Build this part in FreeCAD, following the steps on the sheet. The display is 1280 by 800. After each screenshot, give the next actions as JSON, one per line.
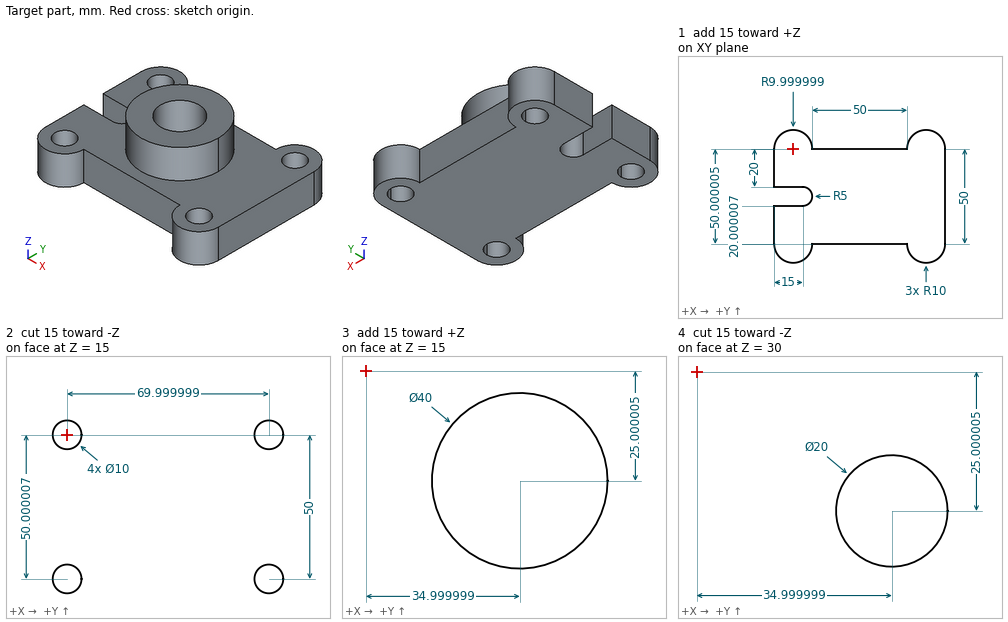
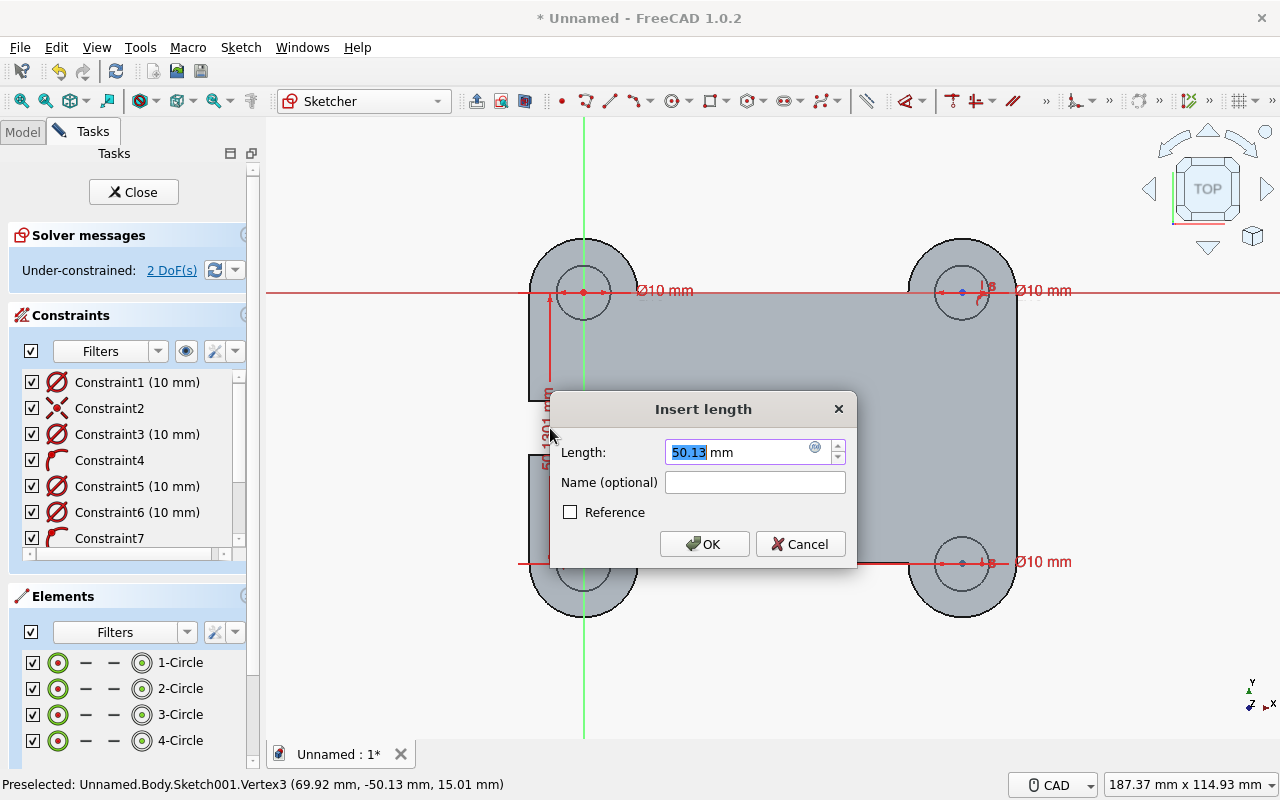
{"action": "type", "text": "50"}
{"action": "key", "text": "Return"}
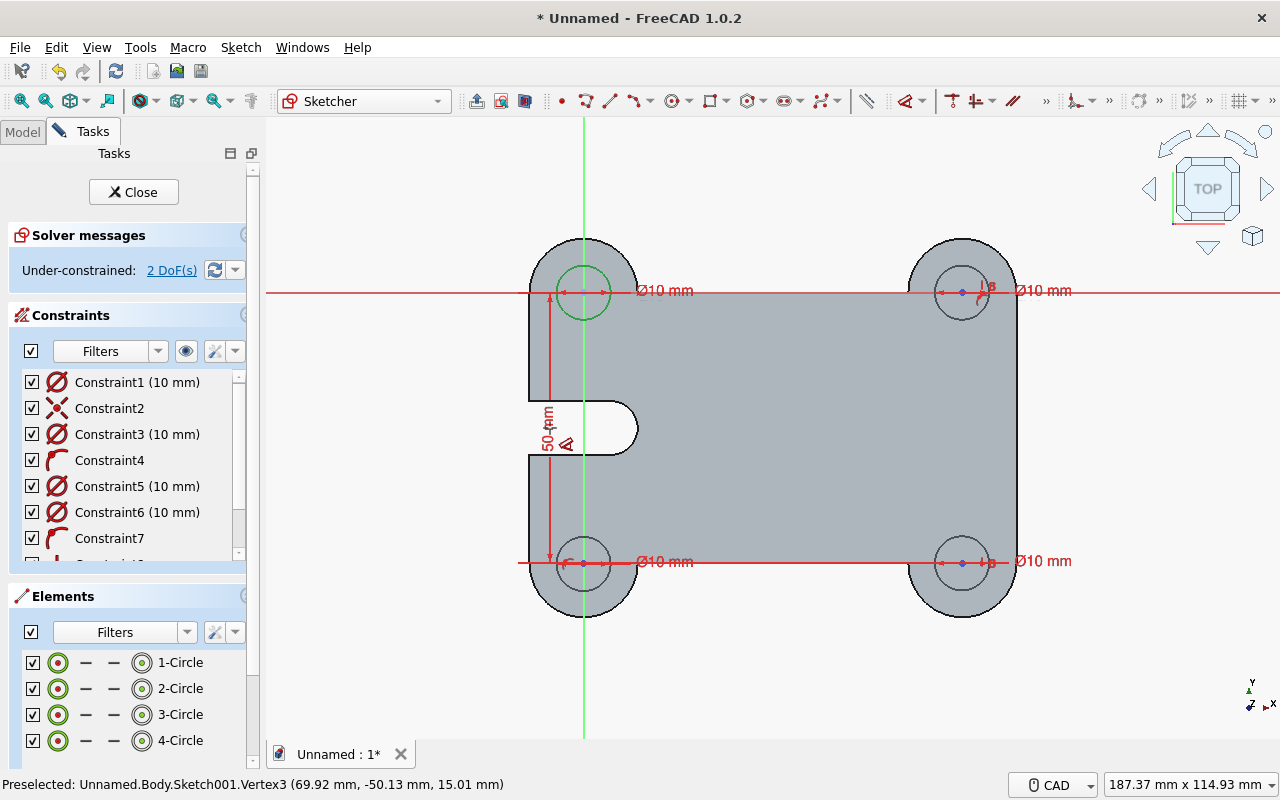
{"action": "left_click", "coordinate": [962, 293]}
{"action": "left_click", "coordinate": [773, 259]}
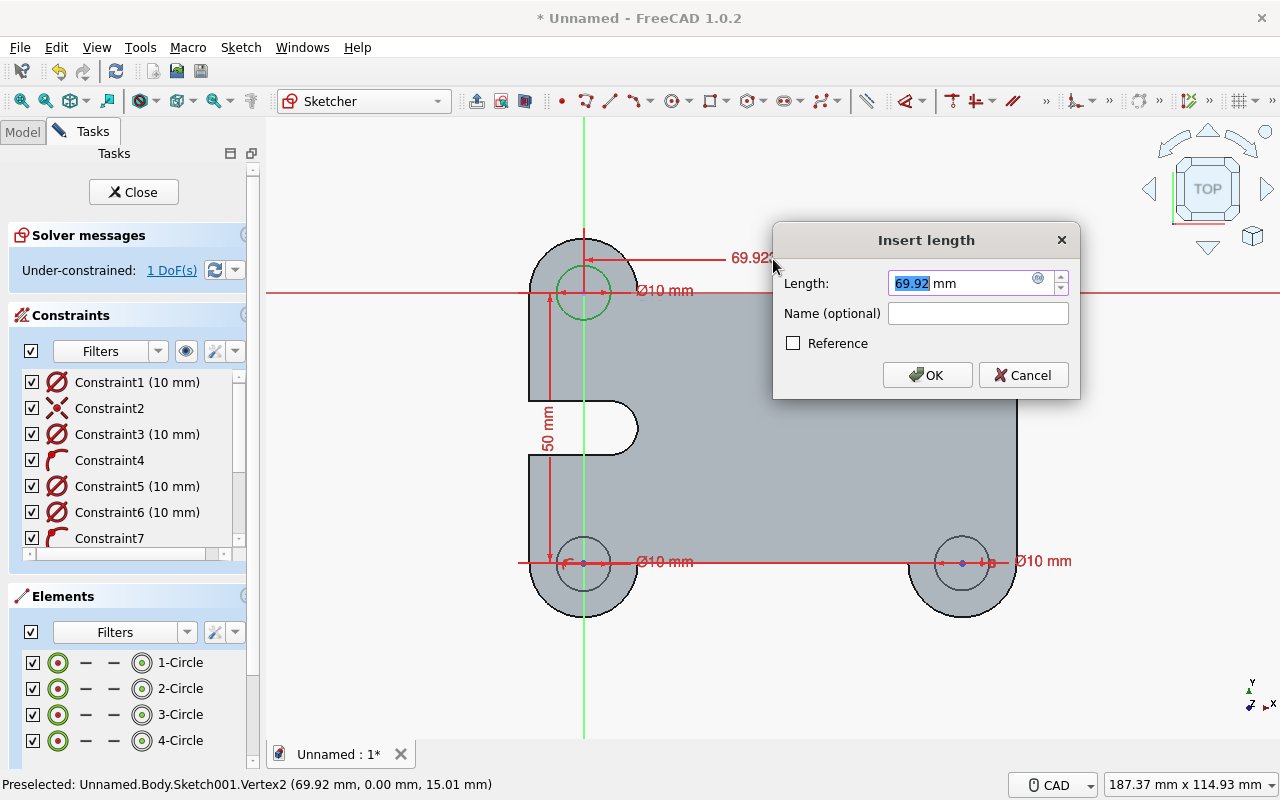
{"action": "type", "text": "69.999999"}
{"action": "key", "text": "Return"}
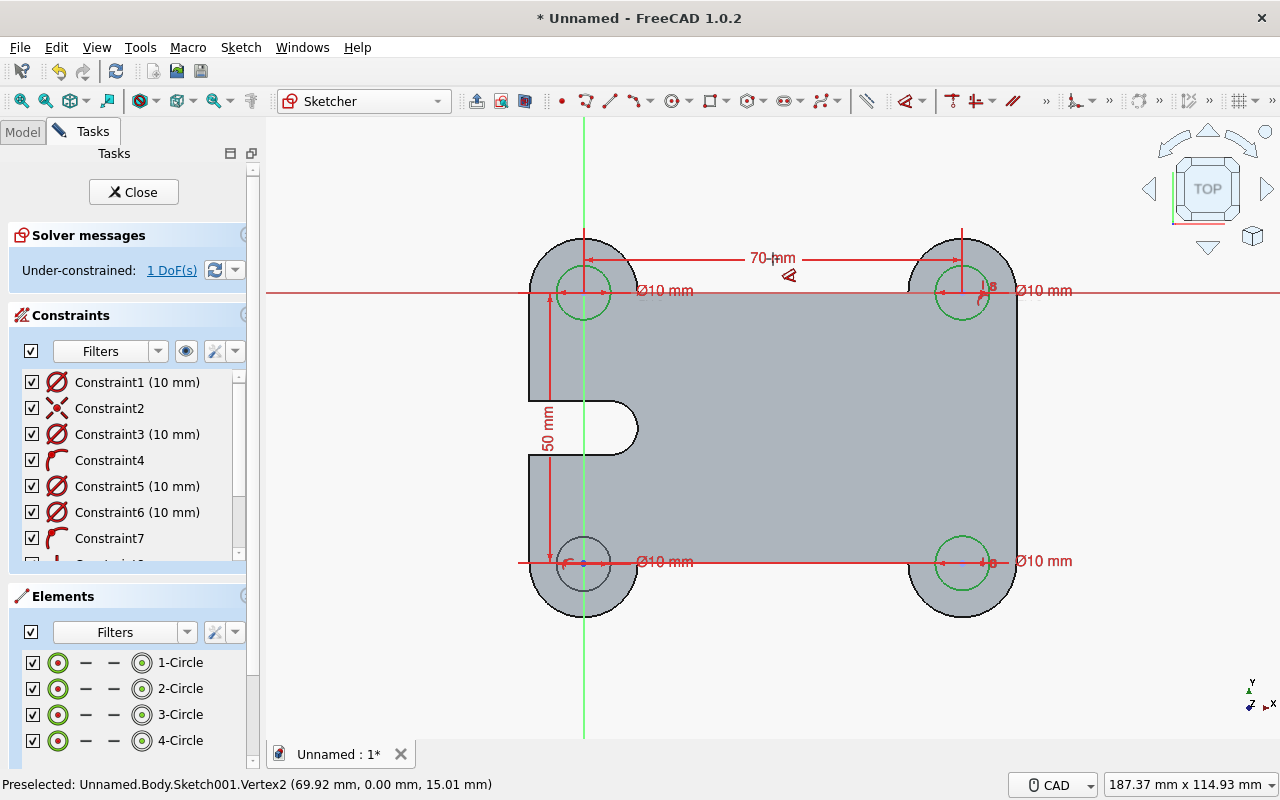
{"action": "left_click", "coordinate": [584, 564]}
{"action": "left_click", "coordinate": [550, 366]}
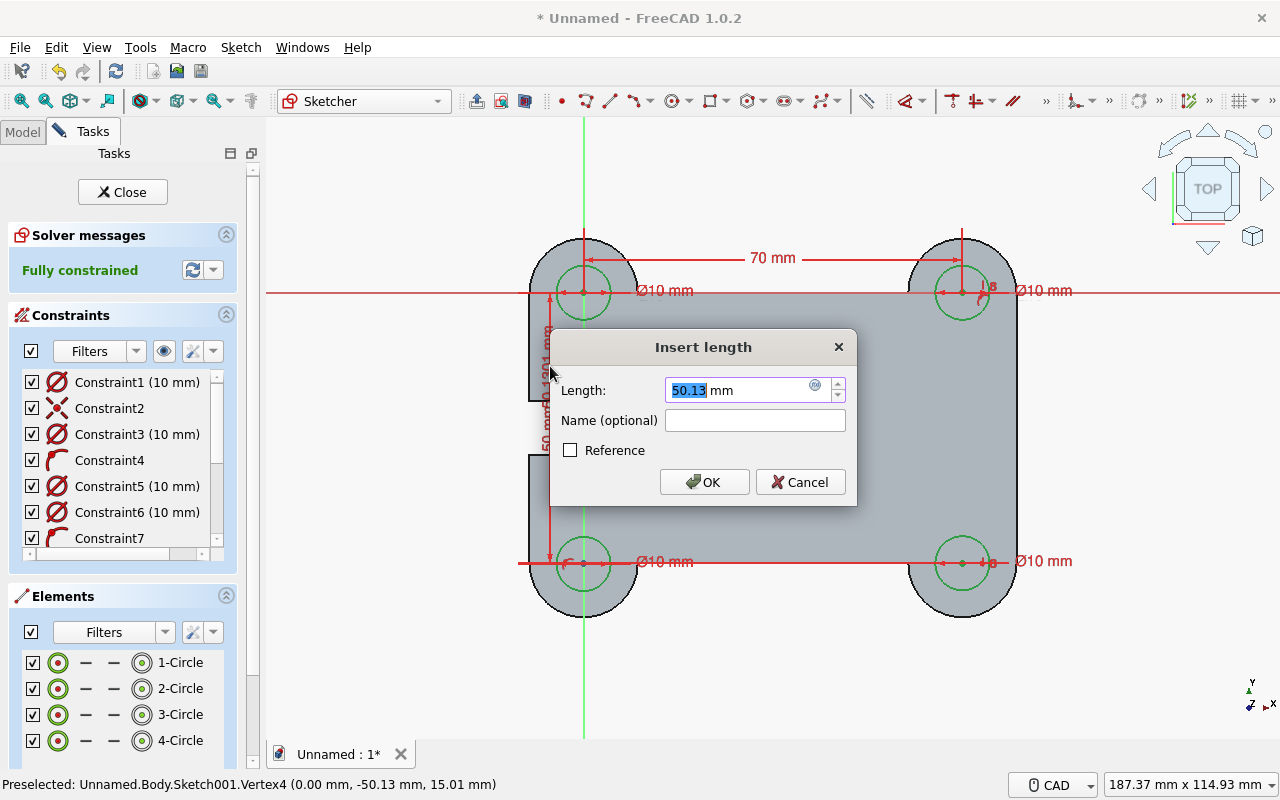
{"action": "type", "text": "50.000007"}
{"action": "key", "text": "Return"}
{"action": "key", "text": "Escape"}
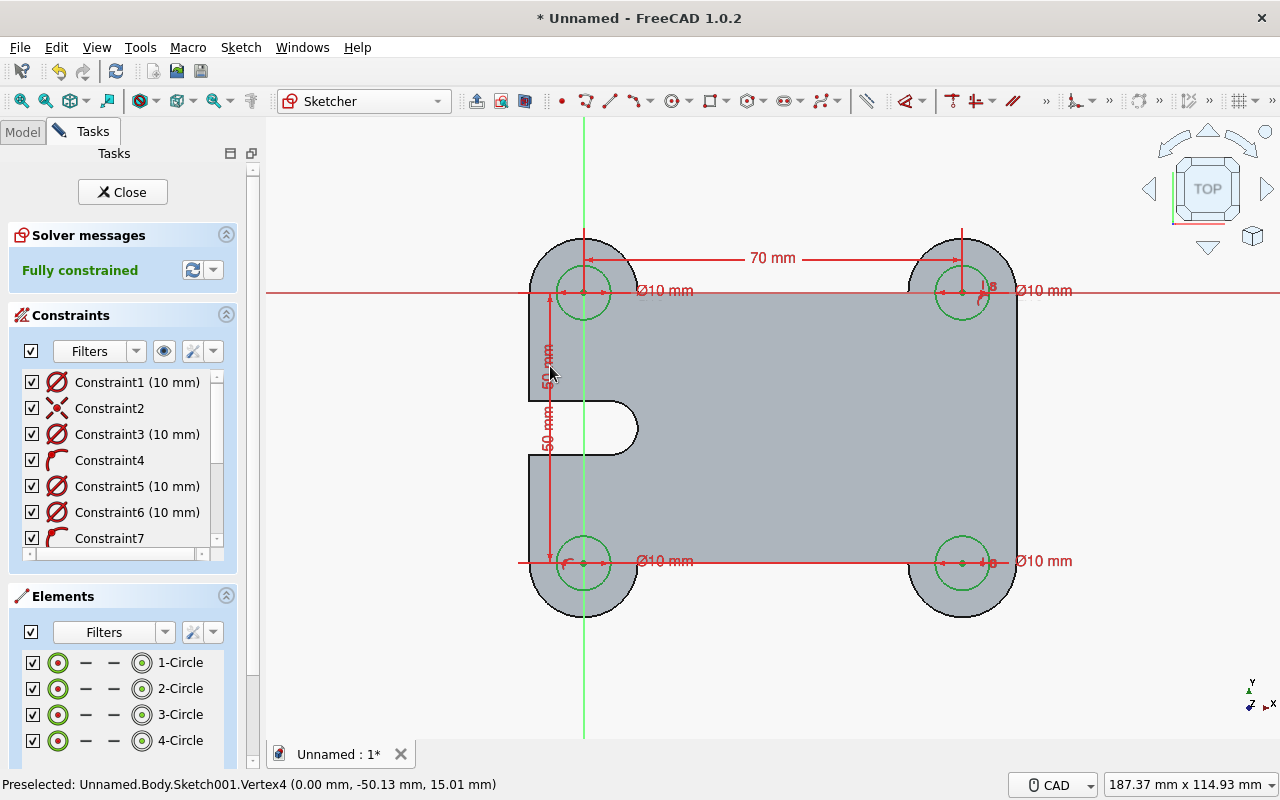
{"action": "left_click", "coordinate": [123, 192]}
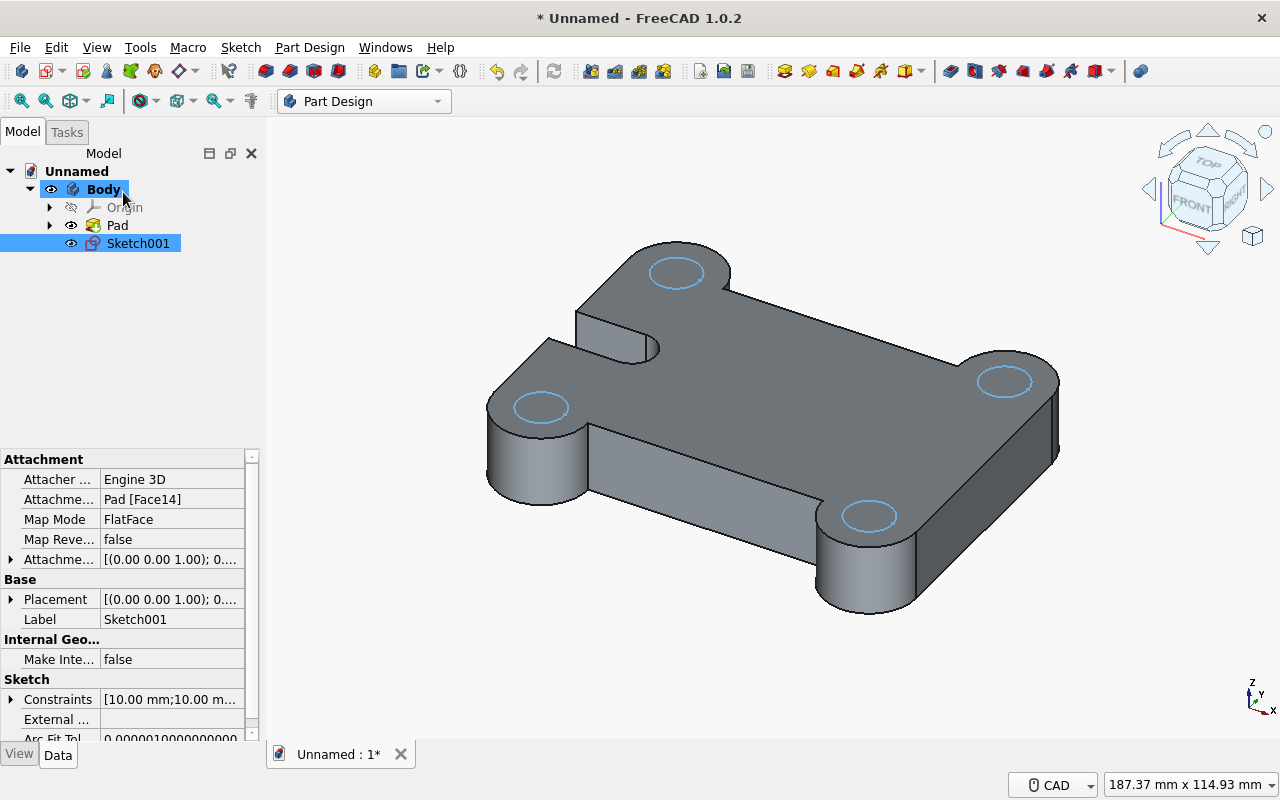
{"action": "left_click", "coordinate": [952, 72]}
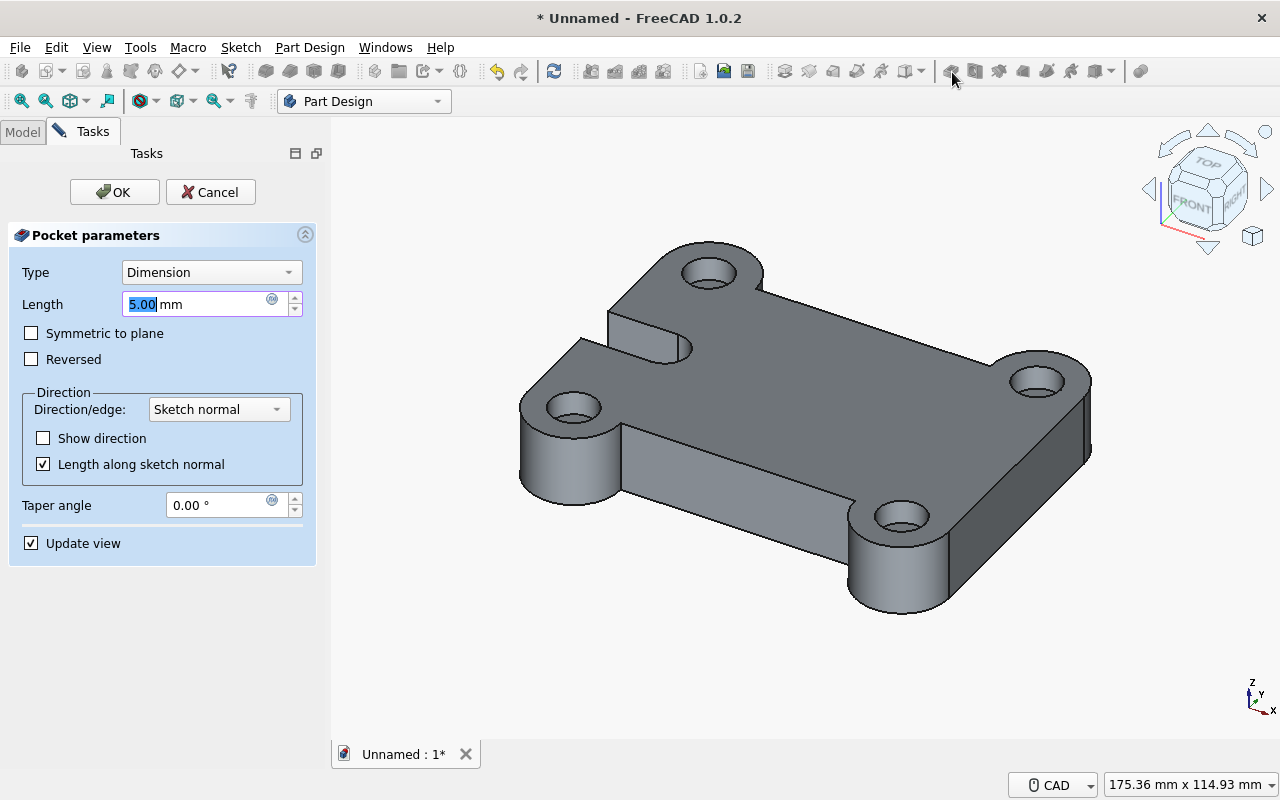
{"action": "type", "text": "15"}
{"action": "key", "text": "Tab"}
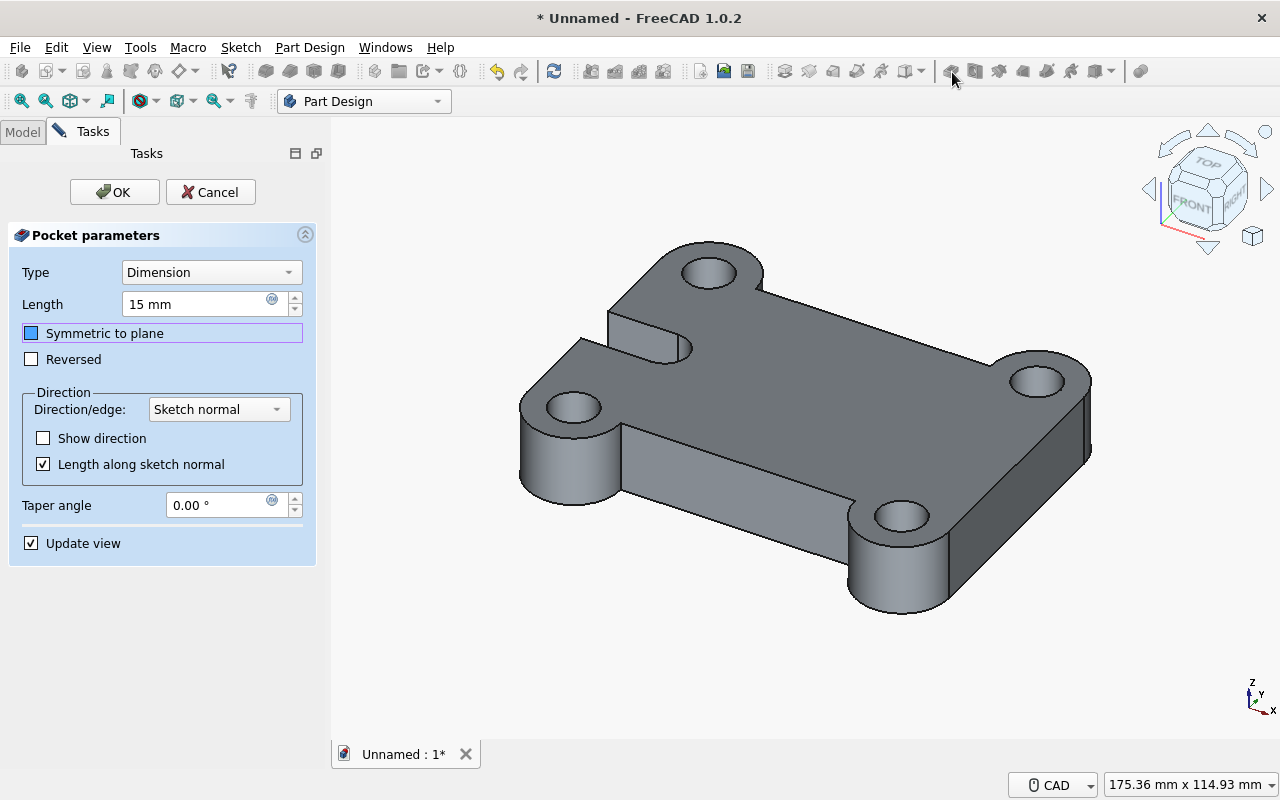
{"action": "left_click", "coordinate": [115, 192]}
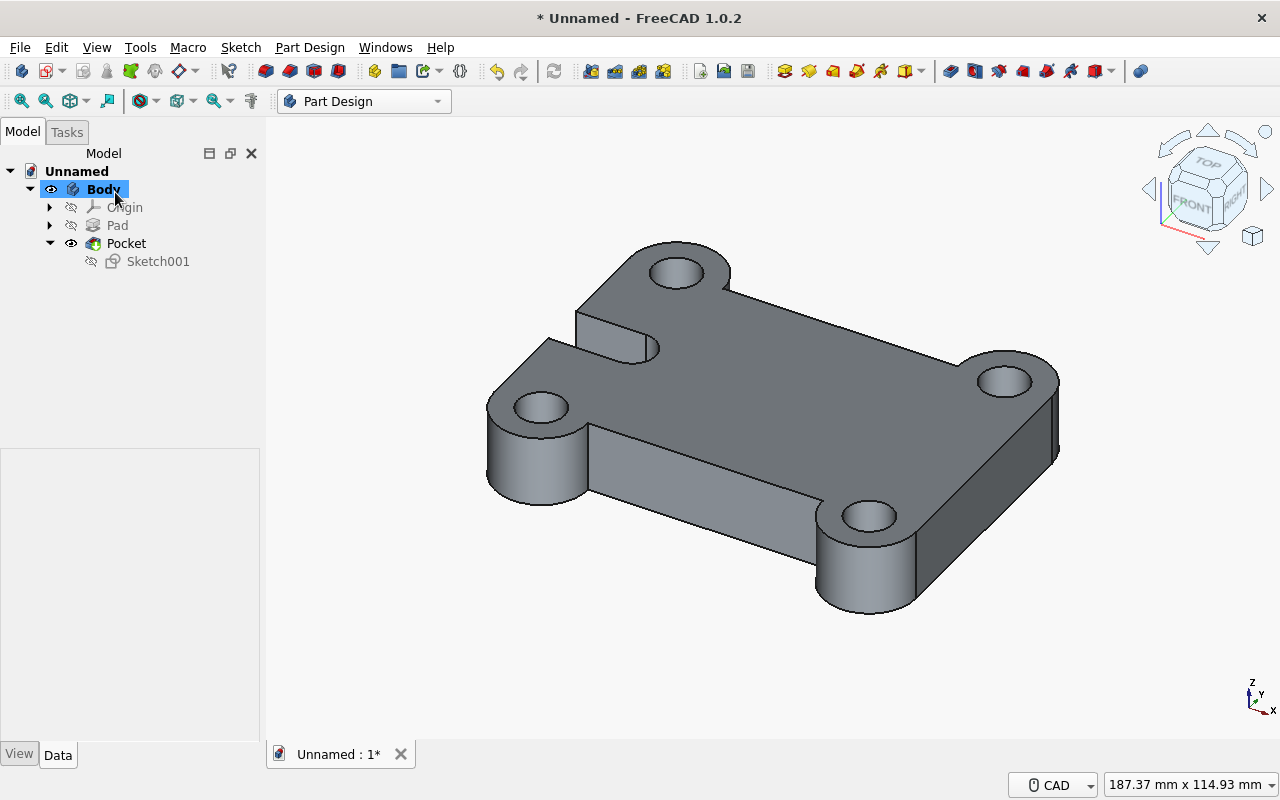
{"action": "left_click", "coordinate": [833, 414]}